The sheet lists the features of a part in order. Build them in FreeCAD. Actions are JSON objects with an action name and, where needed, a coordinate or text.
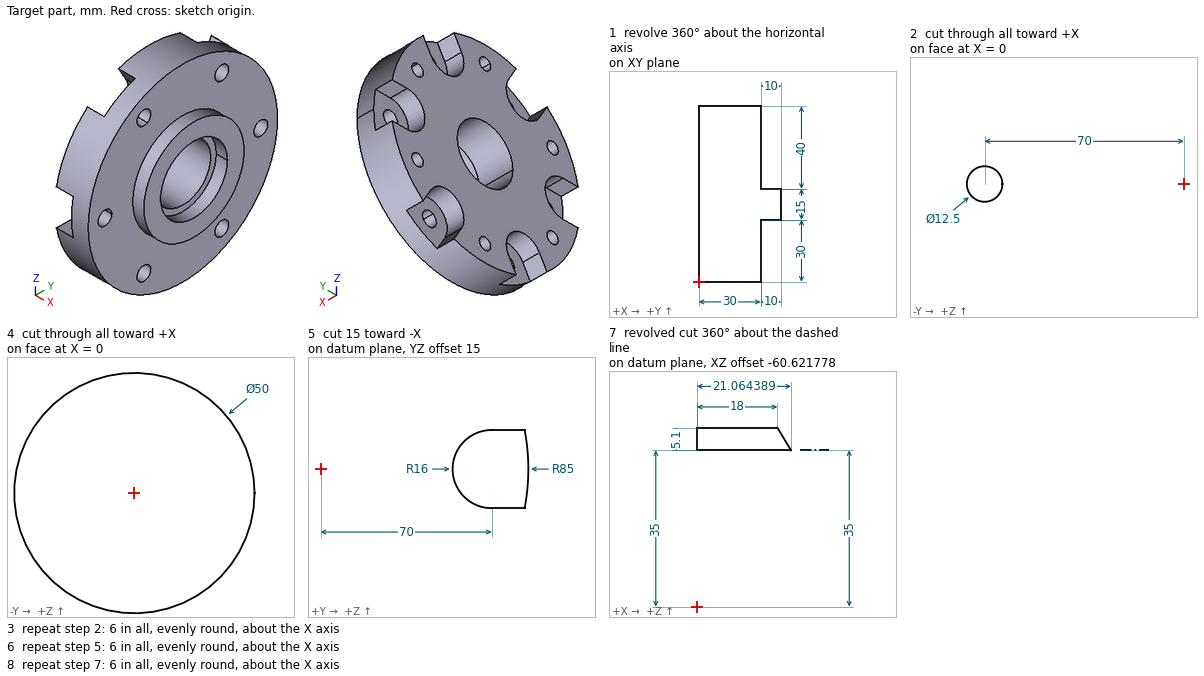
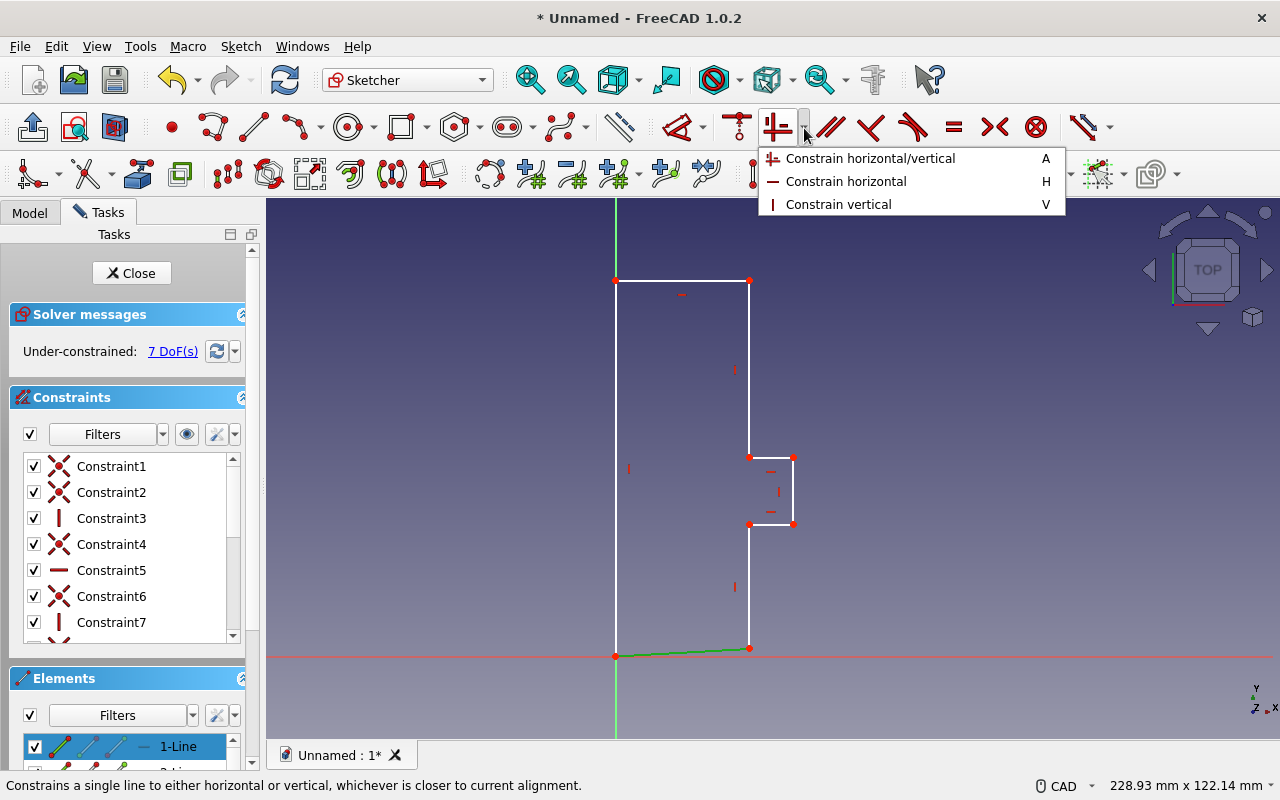
{"action": "left_click", "coordinate": [912, 182]}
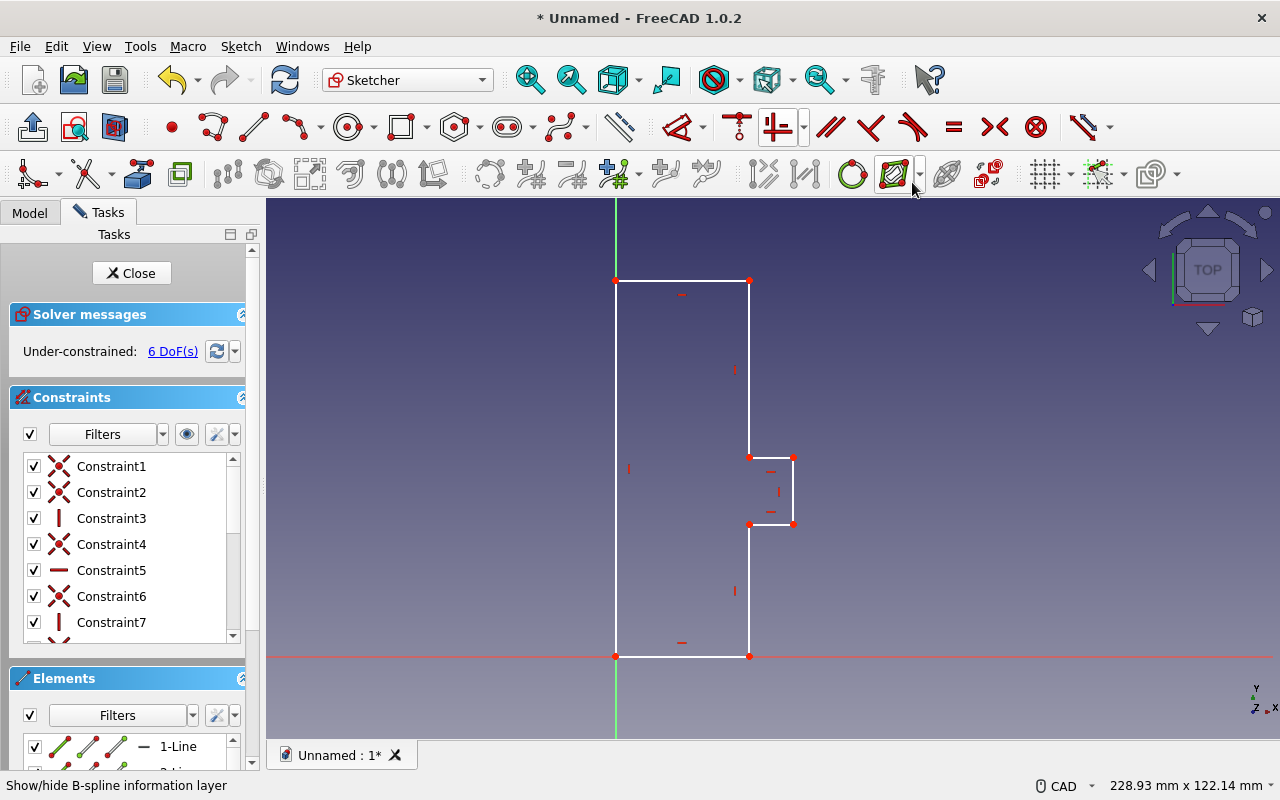
{"action": "left_click", "coordinate": [676, 128]}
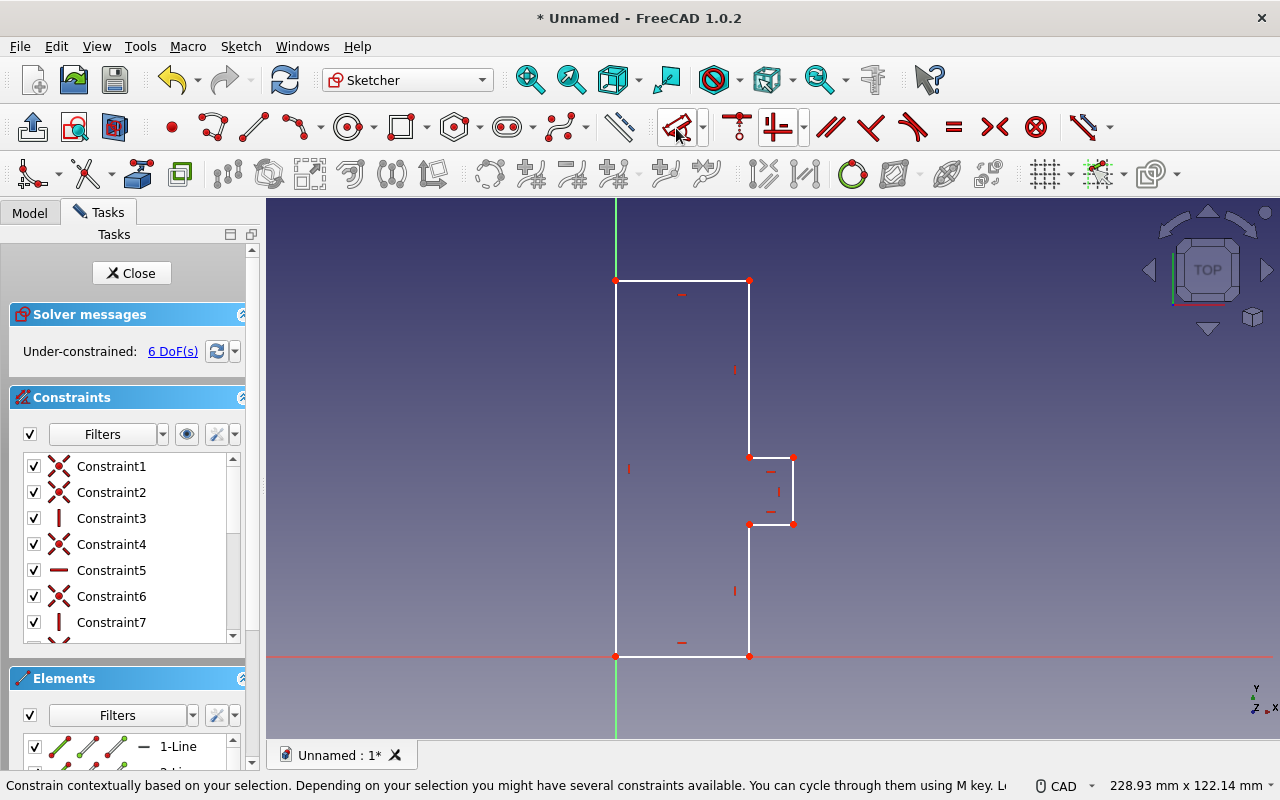
{"action": "left_click", "coordinate": [656, 657]}
{"action": "left_click", "coordinate": [682, 691]}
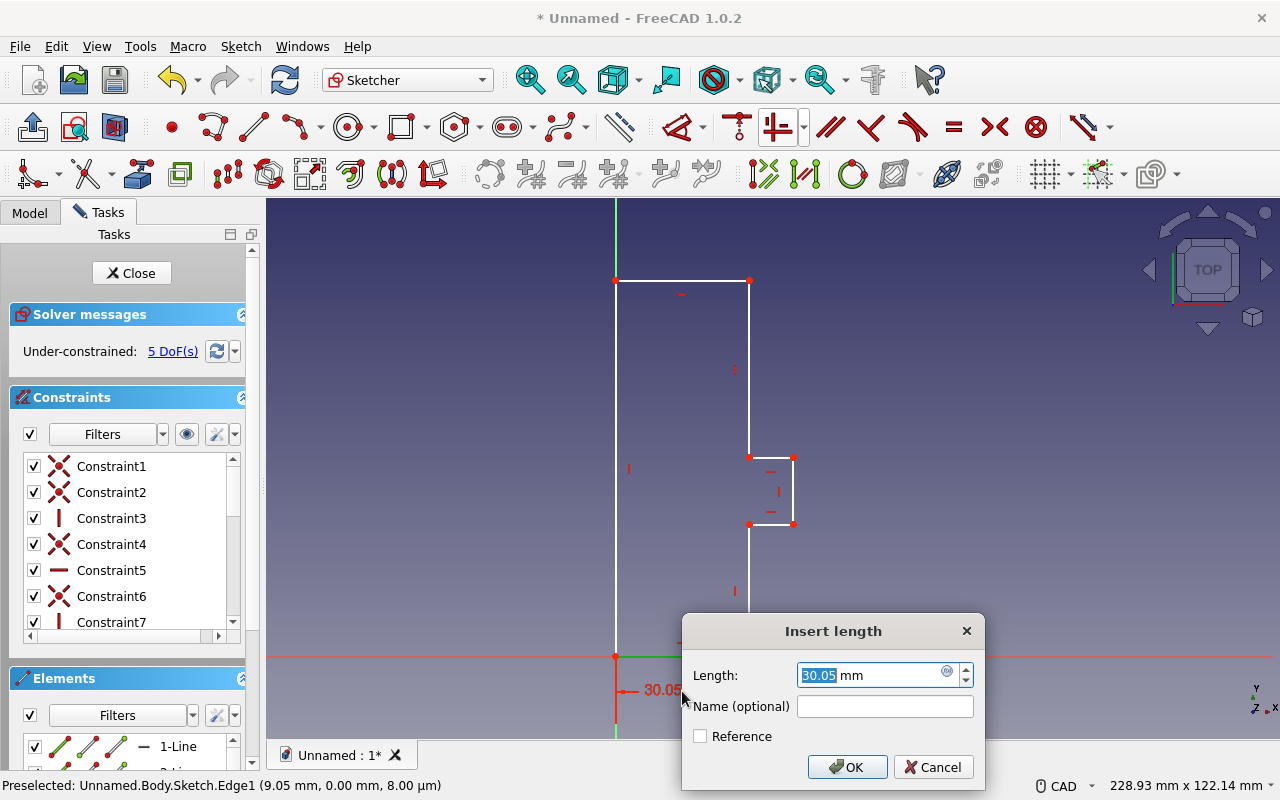
{"action": "type", "text": "30"}
{"action": "key", "text": "Return"}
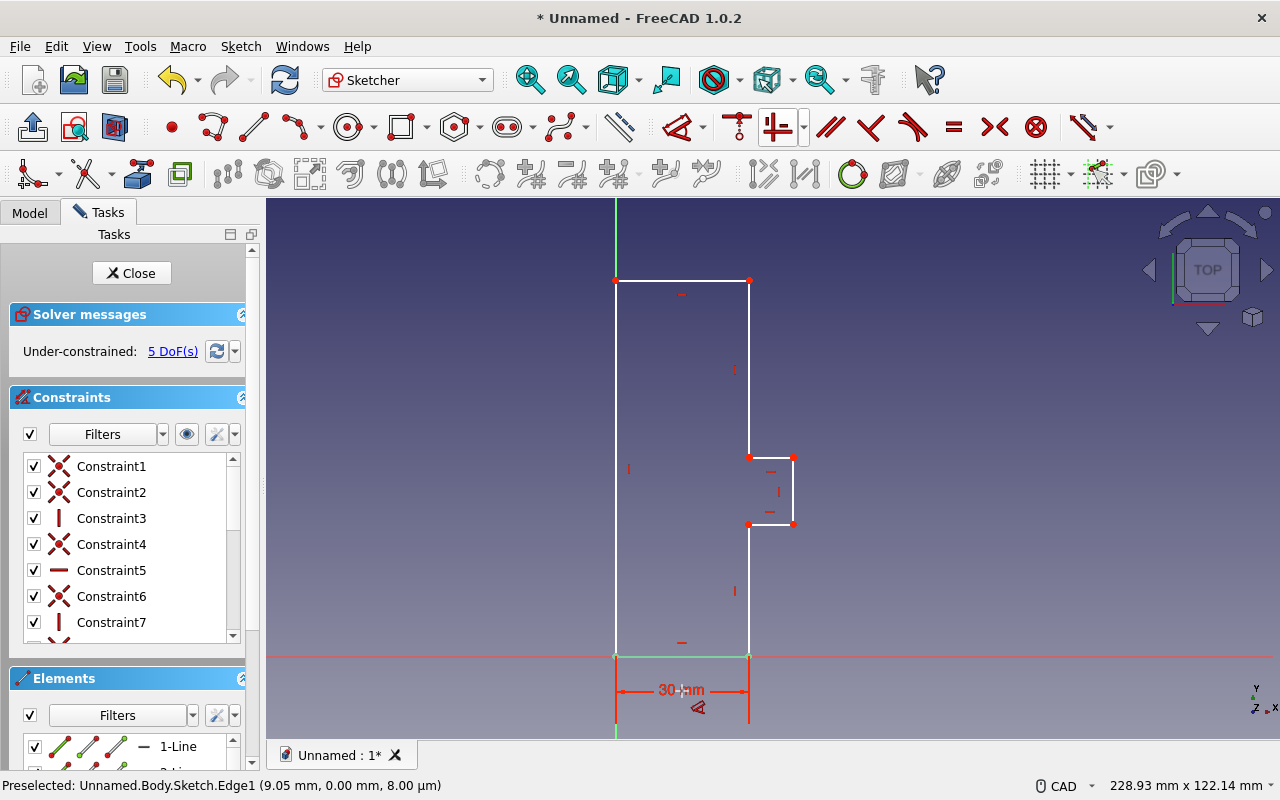
{"action": "left_click", "coordinate": [749, 617]}
{"action": "left_click", "coordinate": [783, 591]}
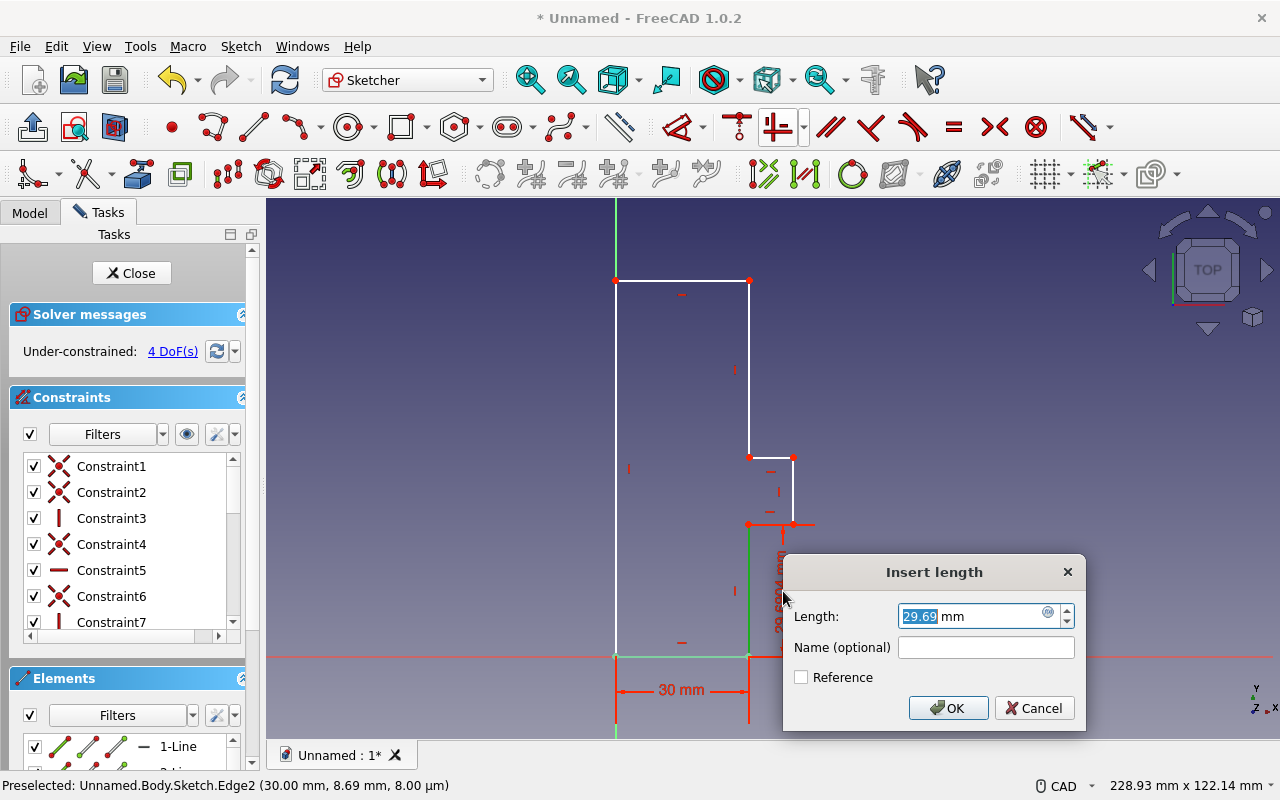
{"action": "type", "text": "30"}
{"action": "key", "text": "Return"}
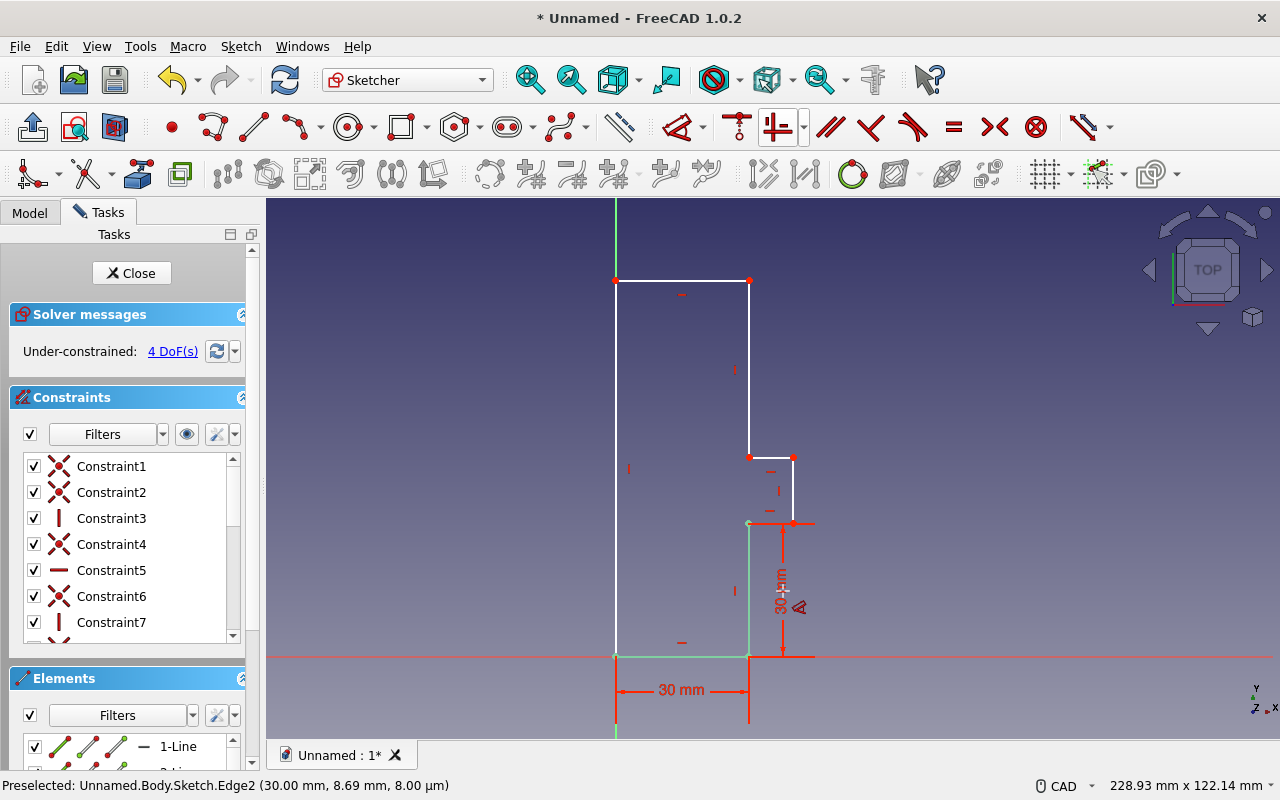
{"action": "left_click", "coordinate": [762, 524]}
{"action": "left_click", "coordinate": [771, 558]}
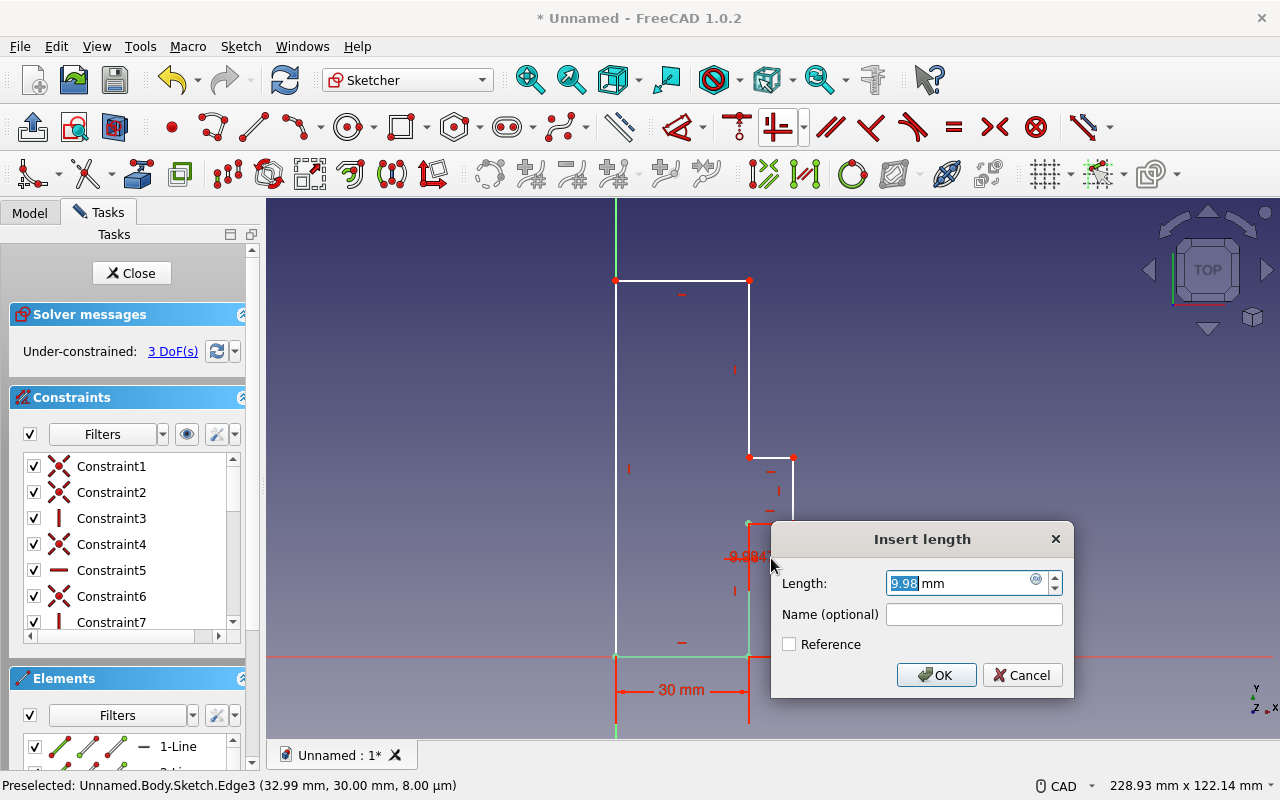
{"action": "type", "text": "10"}
{"action": "key", "text": "Return"}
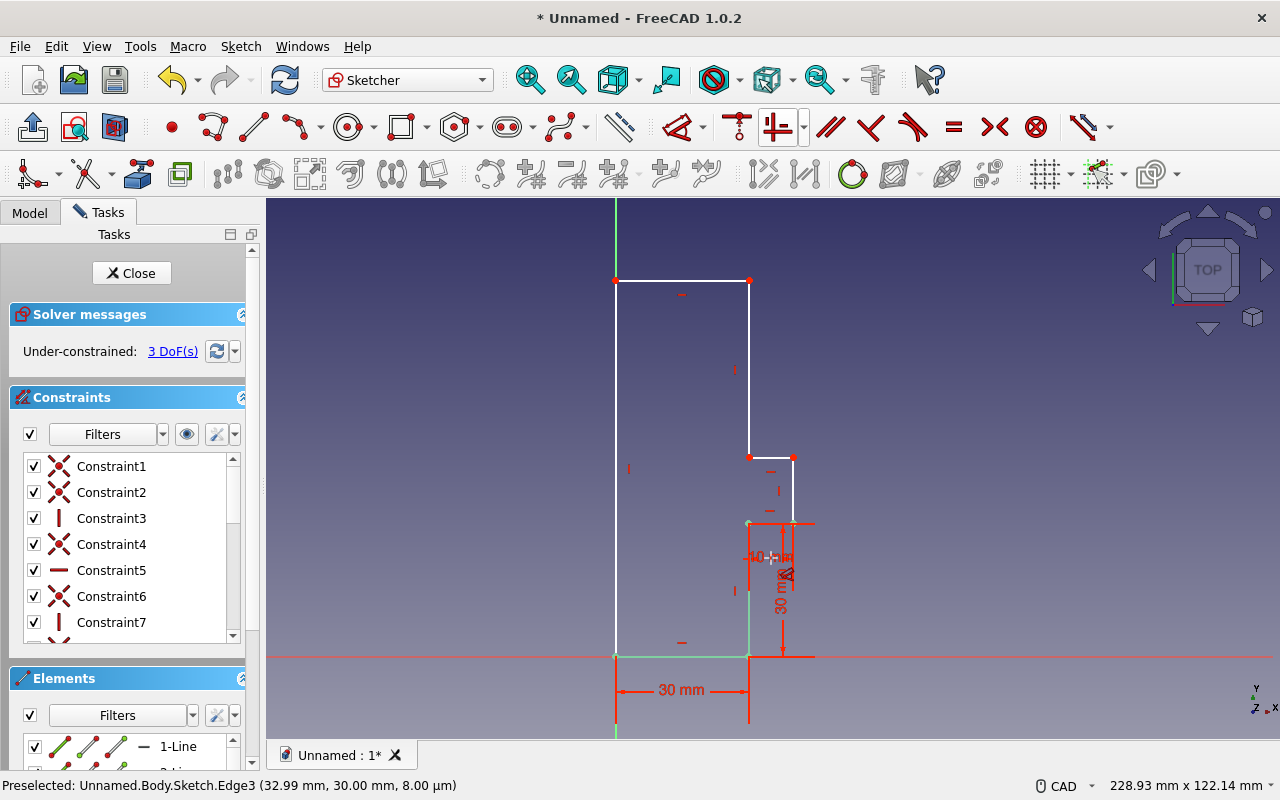
{"action": "left_click", "coordinate": [793, 504]}
{"action": "left_click", "coordinate": [827, 491]}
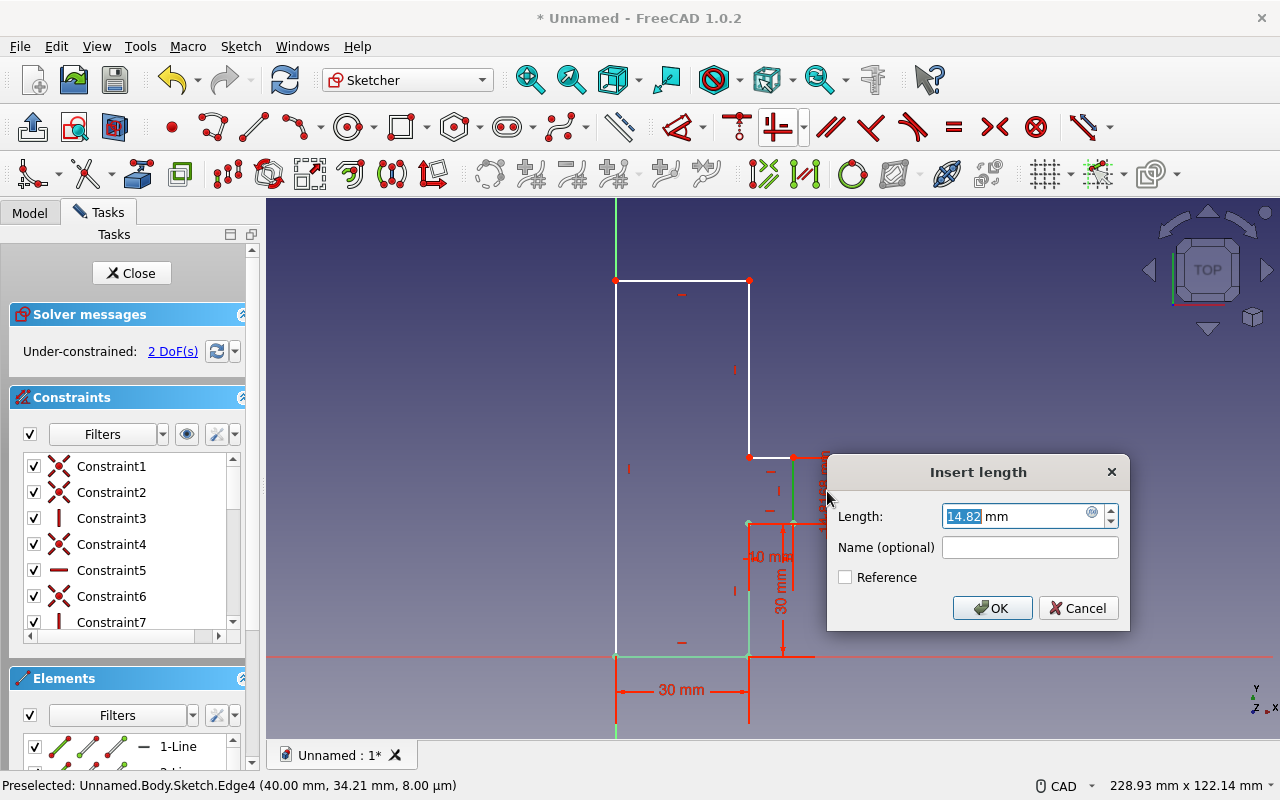
{"action": "type", "text": "15"}
{"action": "key", "text": "Return"}